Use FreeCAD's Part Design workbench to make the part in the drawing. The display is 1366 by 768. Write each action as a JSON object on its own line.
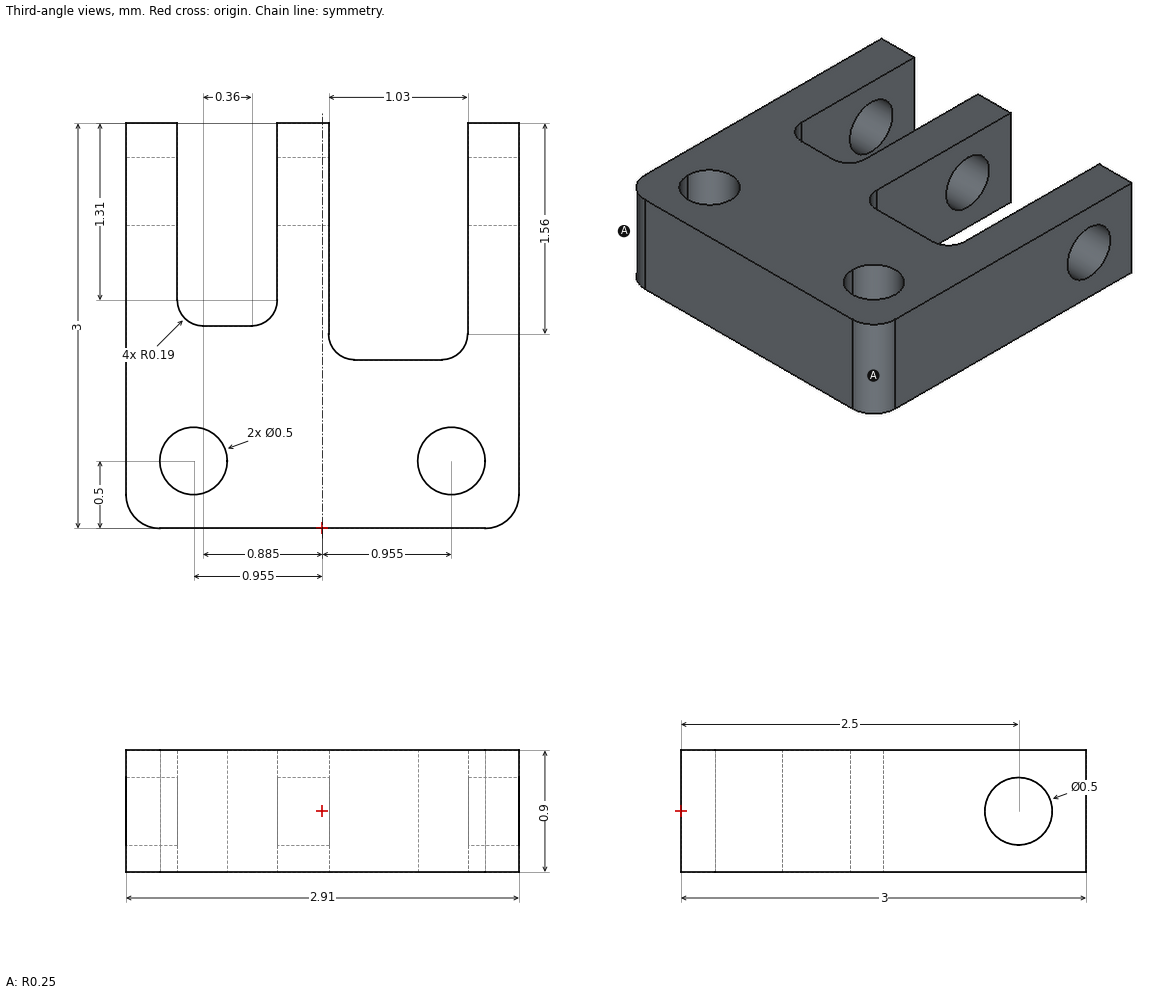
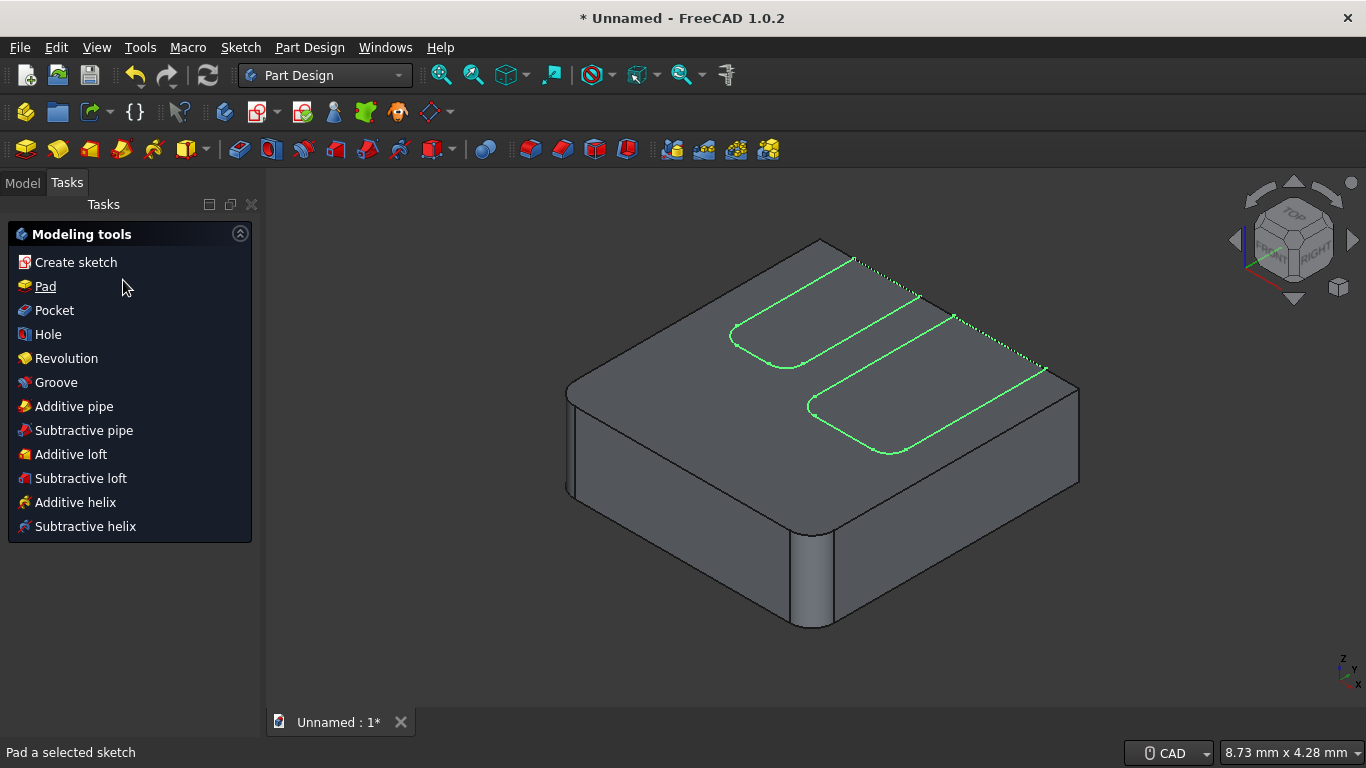
{"action": "left_click", "coordinate": [240, 150]}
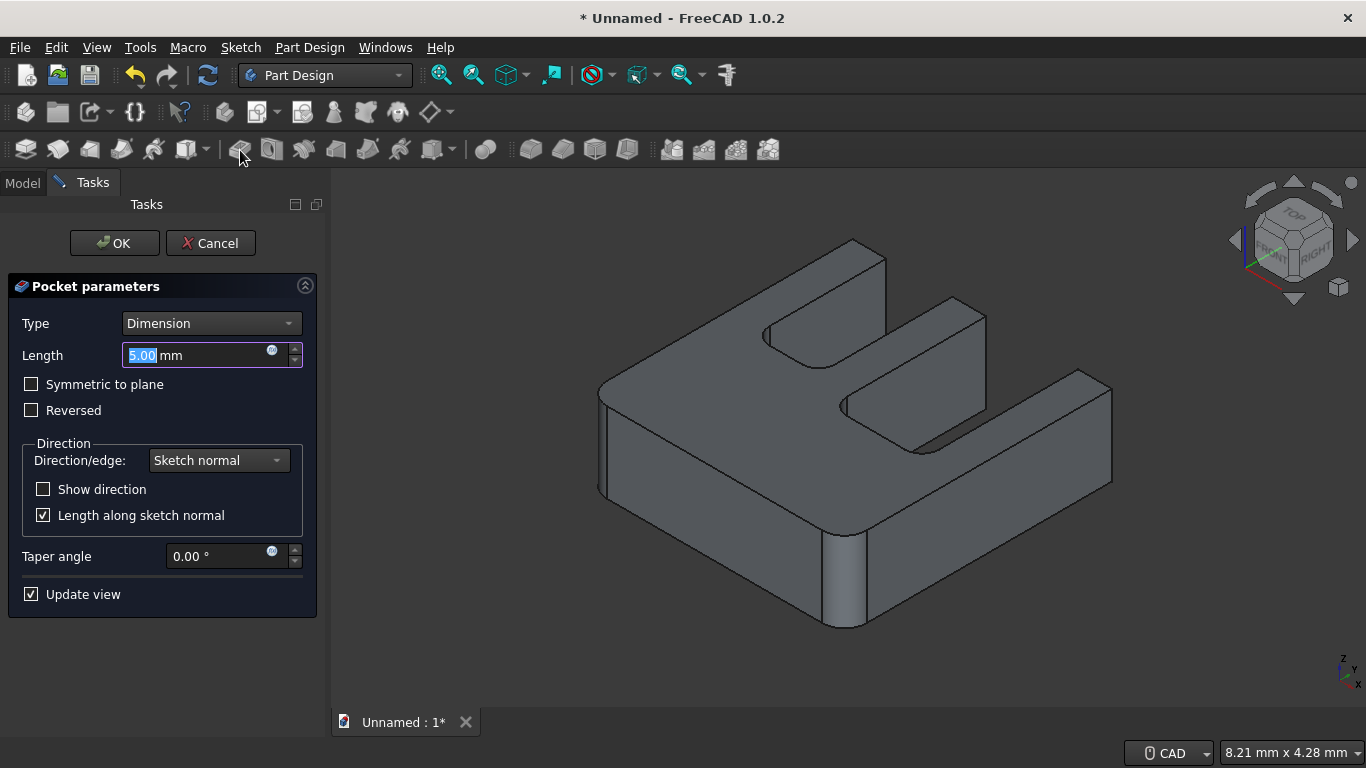
{"action": "type", "text": "3"}
{"action": "key", "text": "Tab"}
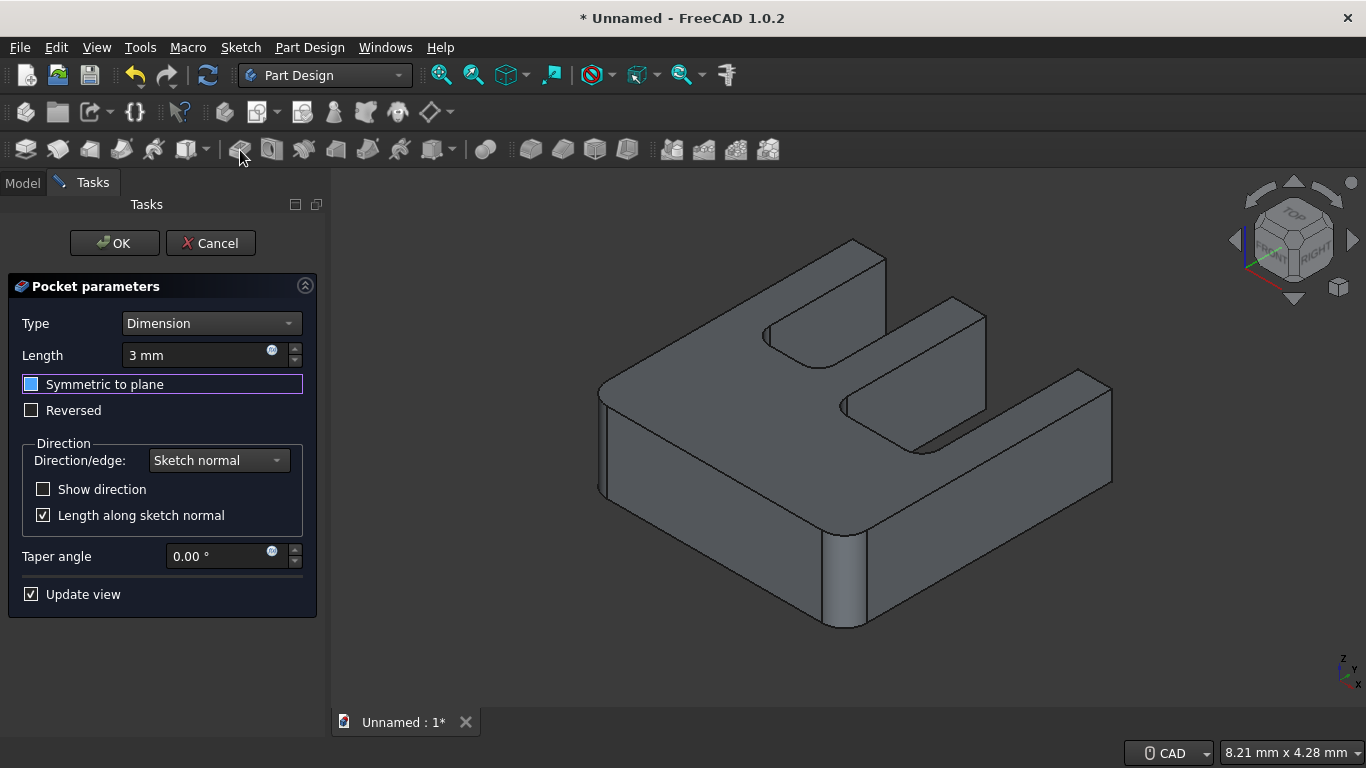
{"action": "left_click", "coordinate": [115, 243]}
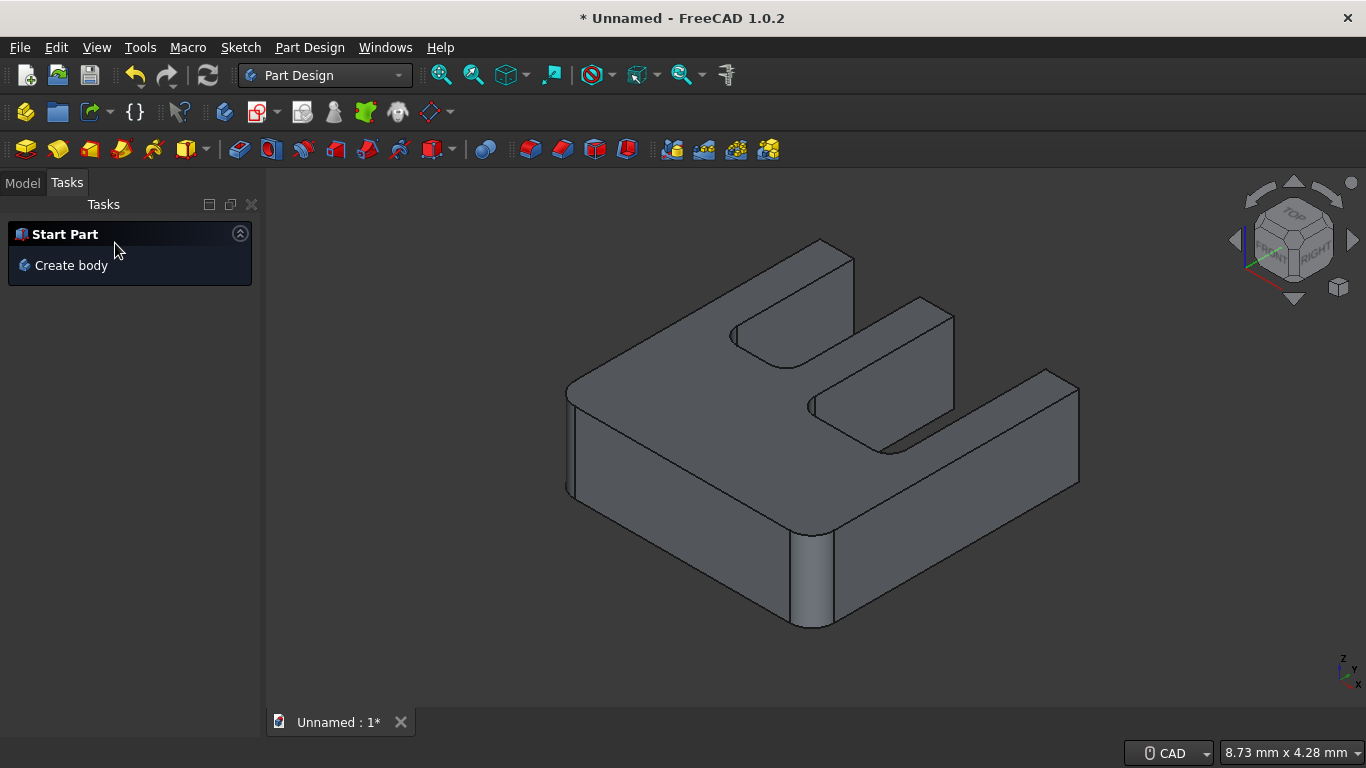
{"action": "left_click", "coordinate": [703, 413]}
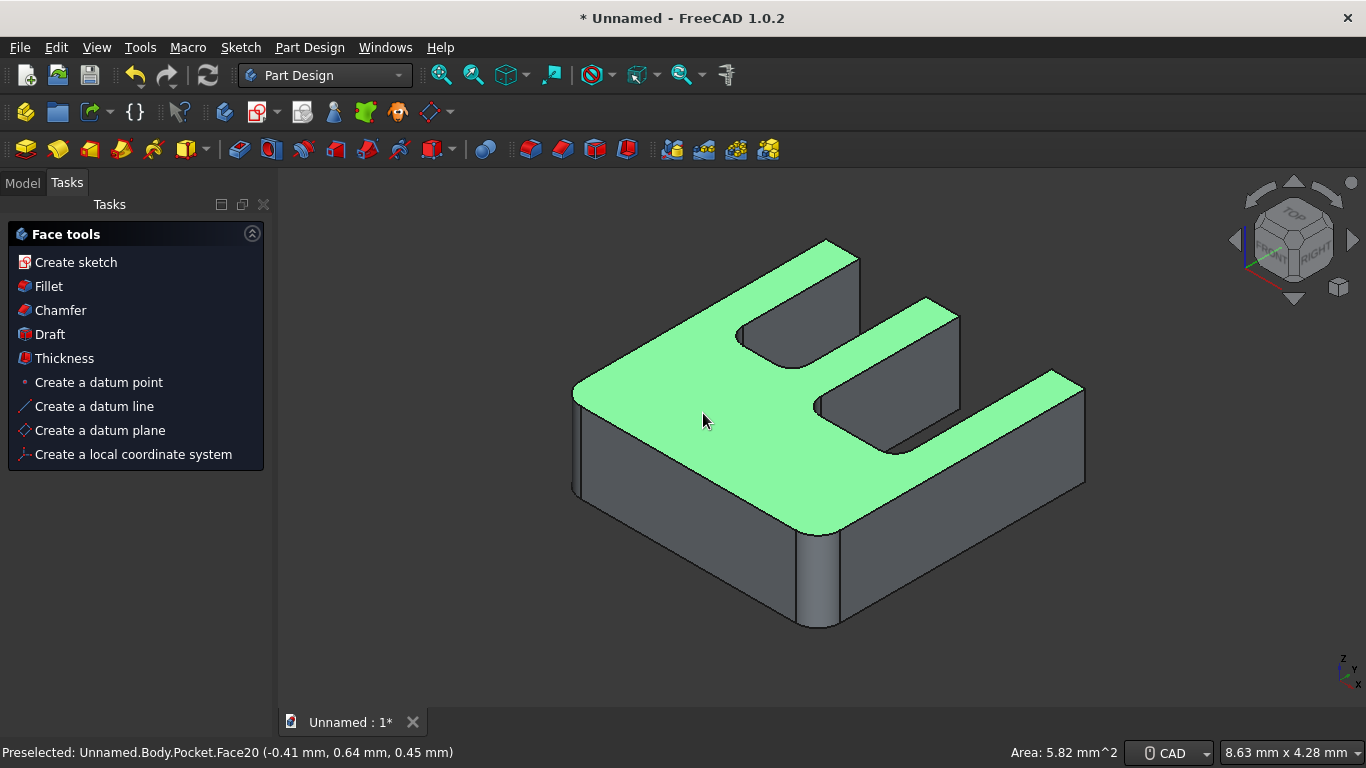
{"action": "left_click", "coordinate": [258, 112]}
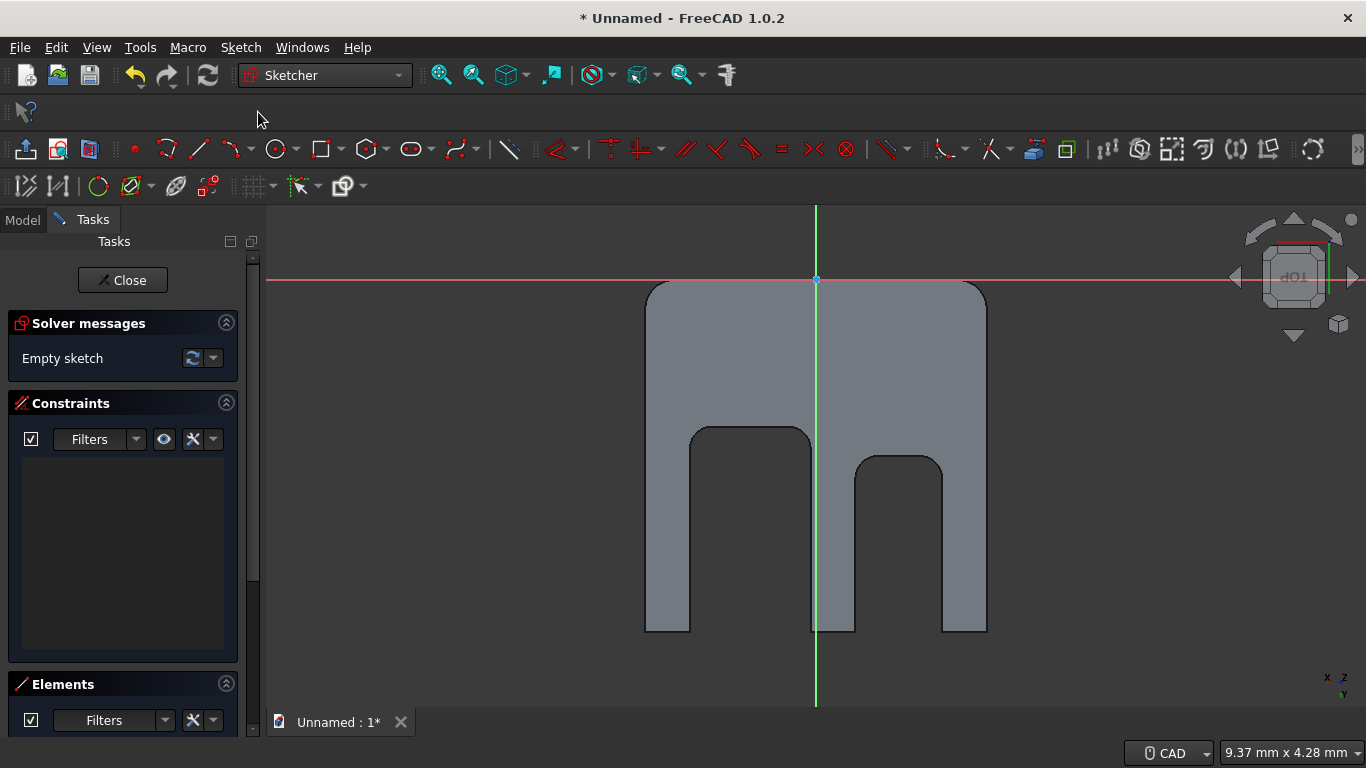
{"action": "scroll", "coordinate": [872, 233], "scroll_direction": "up", "scroll_amount": 4}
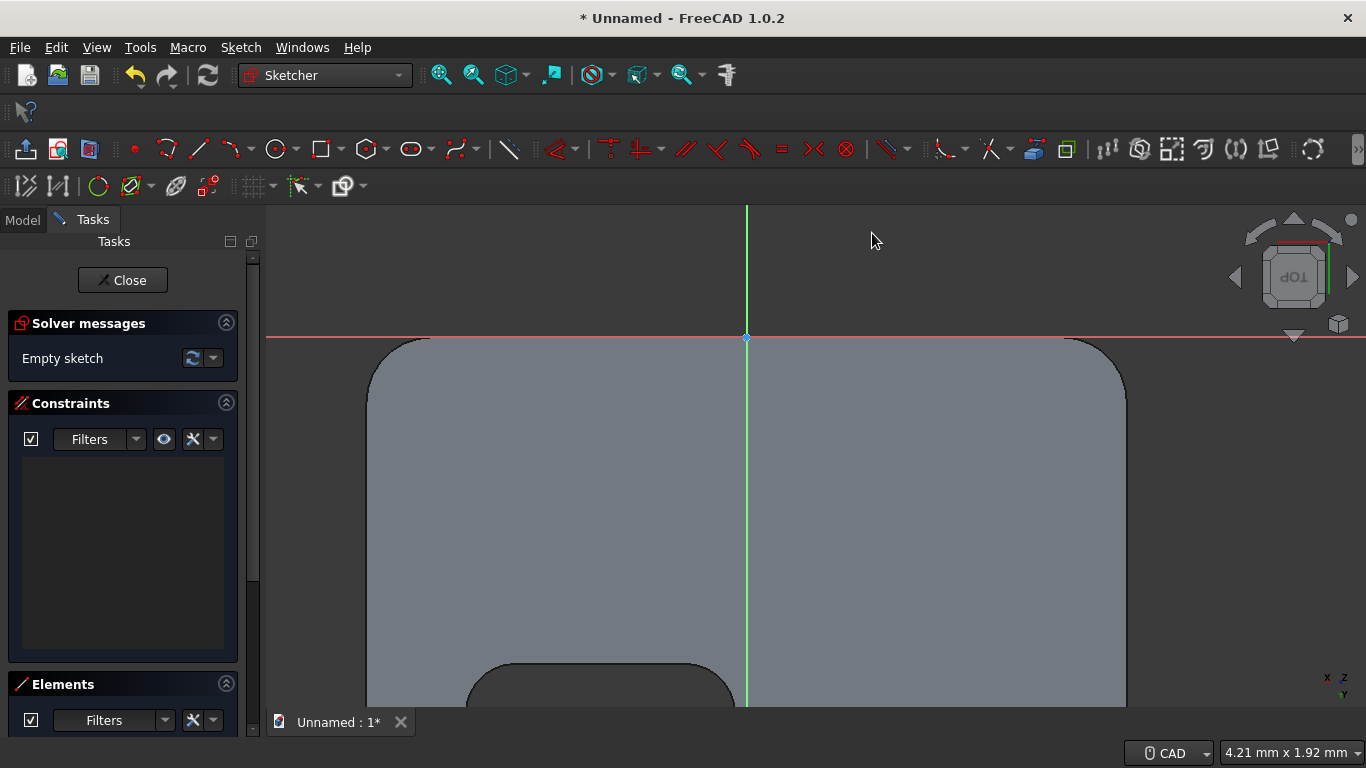
{"action": "key", "text": "g c"}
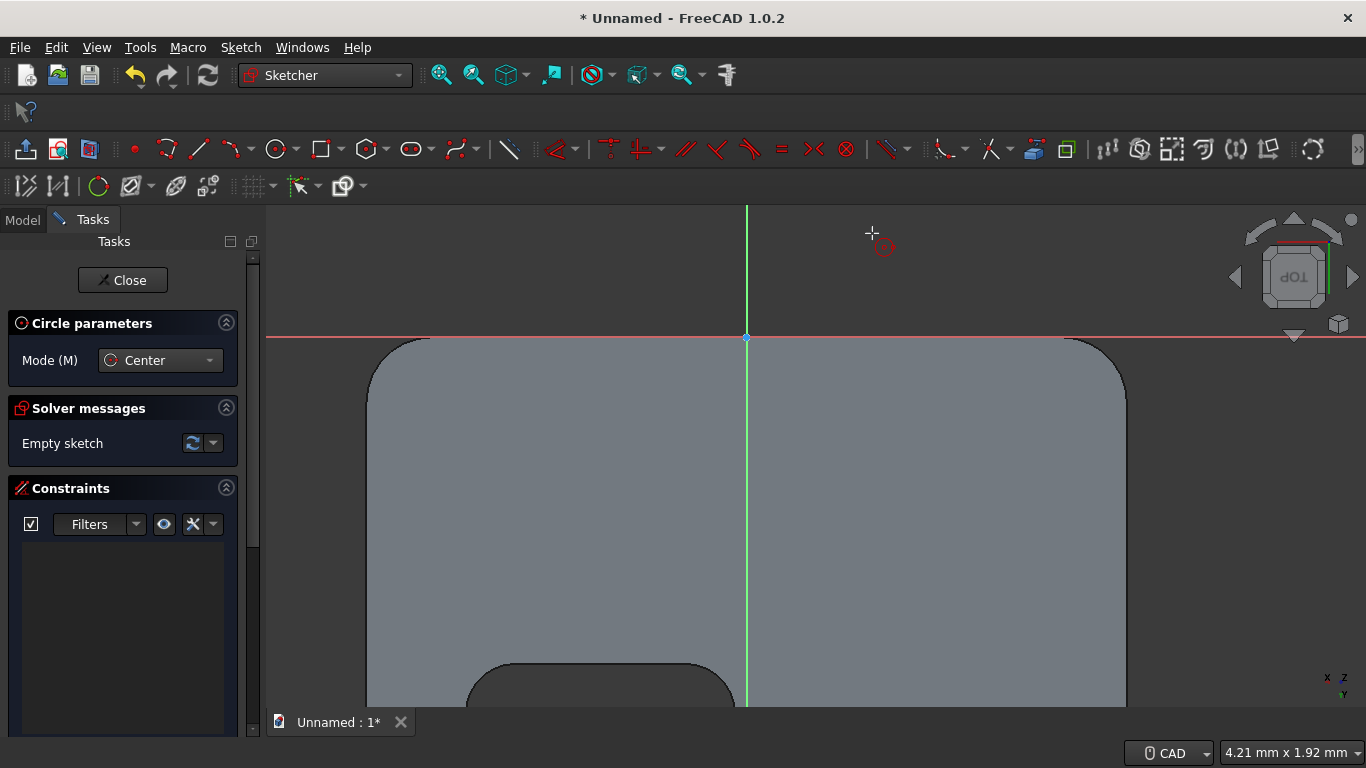
{"action": "left_click", "coordinate": [996, 468]}
{"action": "left_click", "coordinate": [1042, 422]}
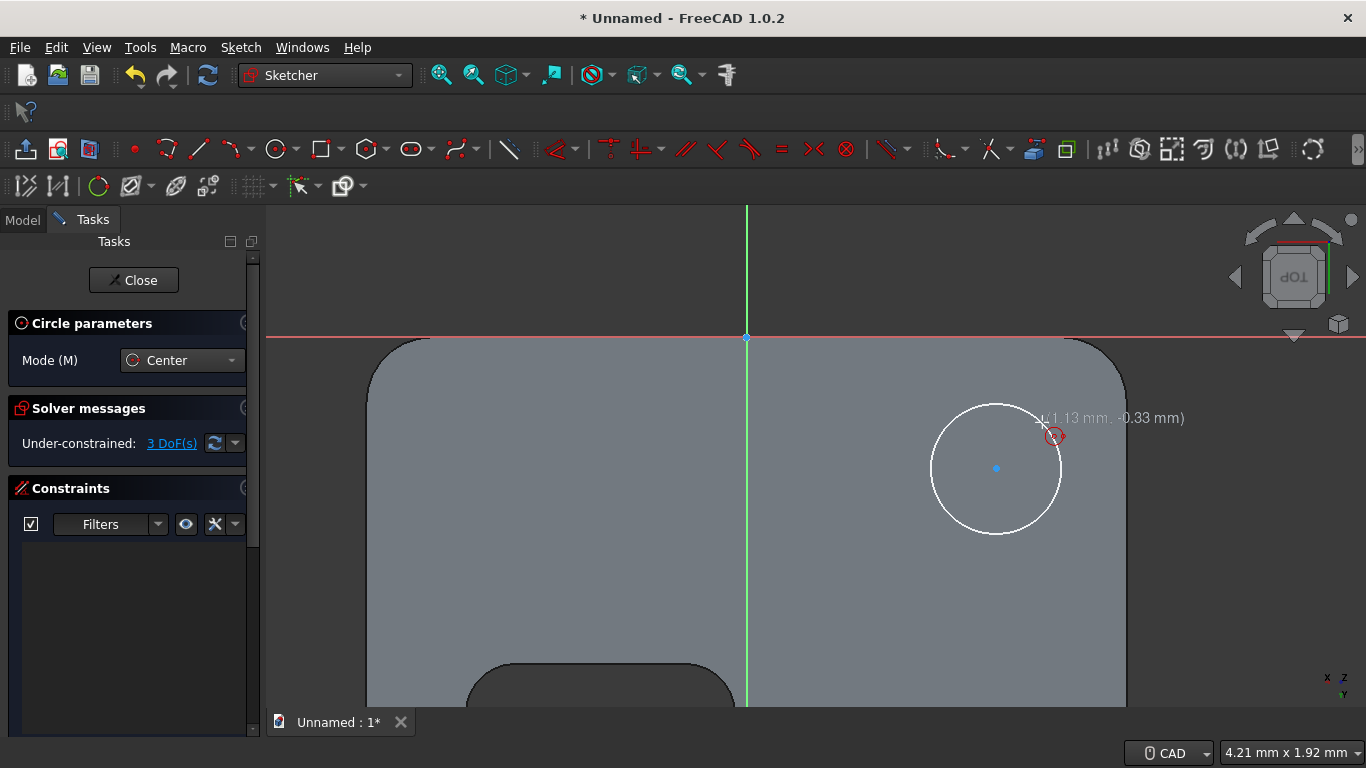
{"action": "left_click", "coordinate": [497, 468]}
{"action": "left_click", "coordinate": [543, 422]}
{"action": "key", "text": "Escape"}